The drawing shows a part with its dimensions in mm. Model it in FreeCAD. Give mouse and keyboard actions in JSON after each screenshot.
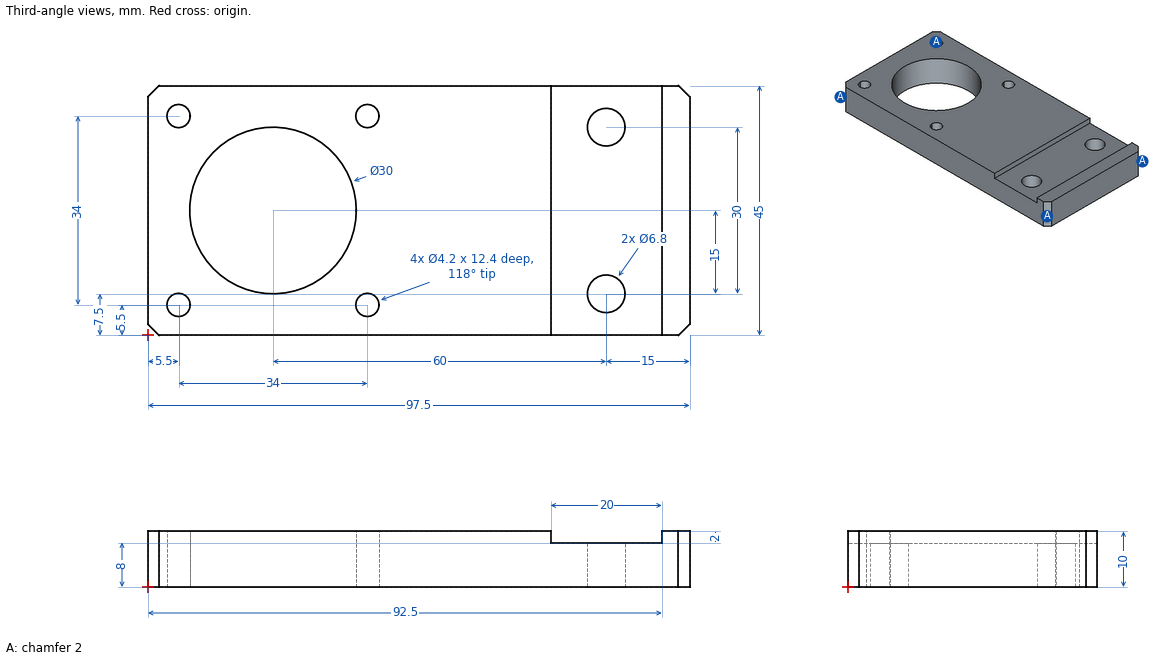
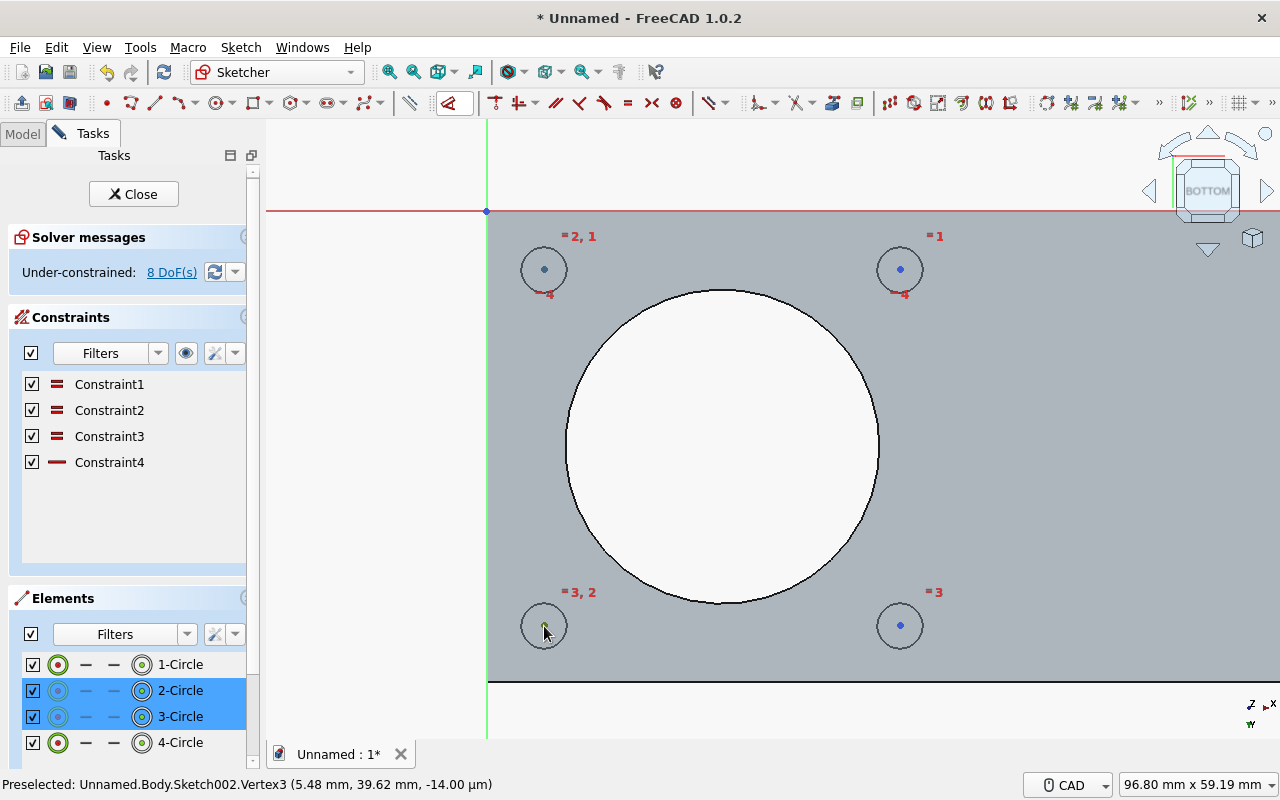
{"action": "left_click", "coordinate": [538, 104]}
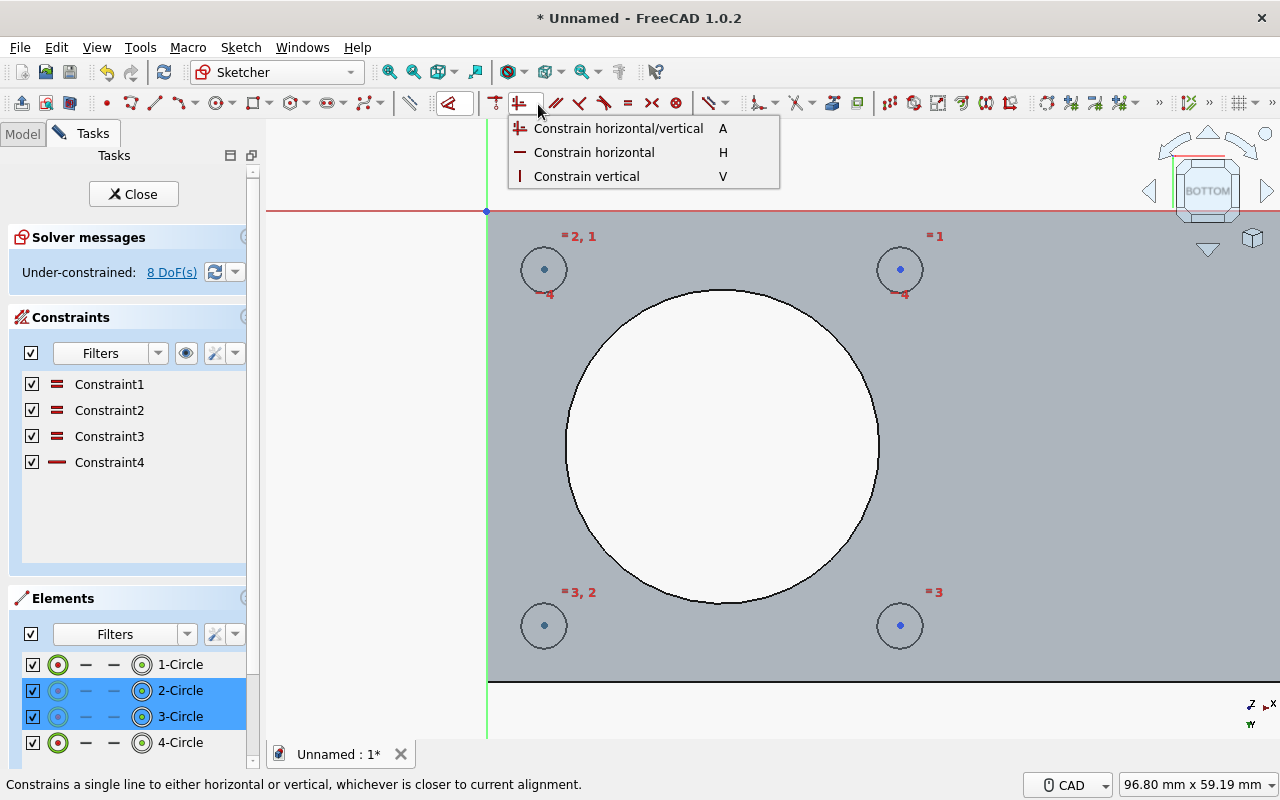
{"action": "left_click", "coordinate": [644, 176]}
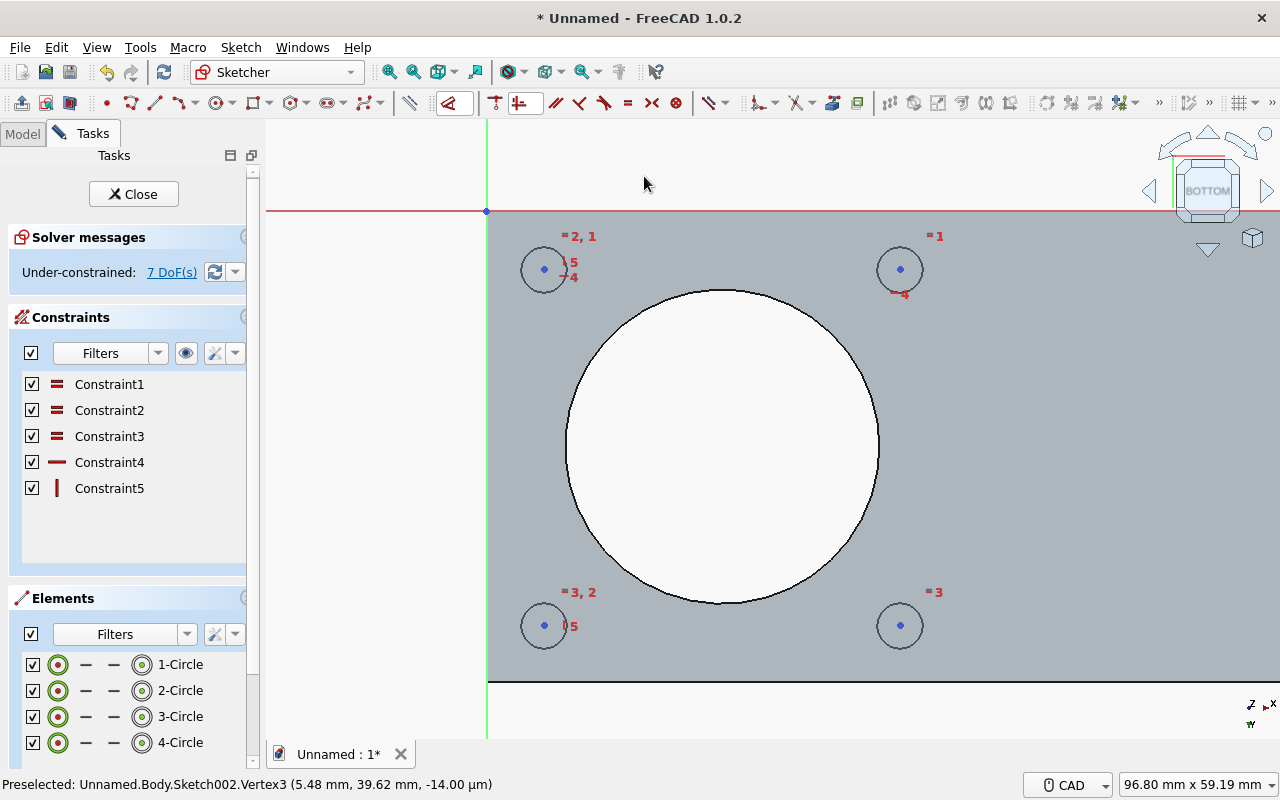
{"action": "left_click", "coordinate": [900, 270]}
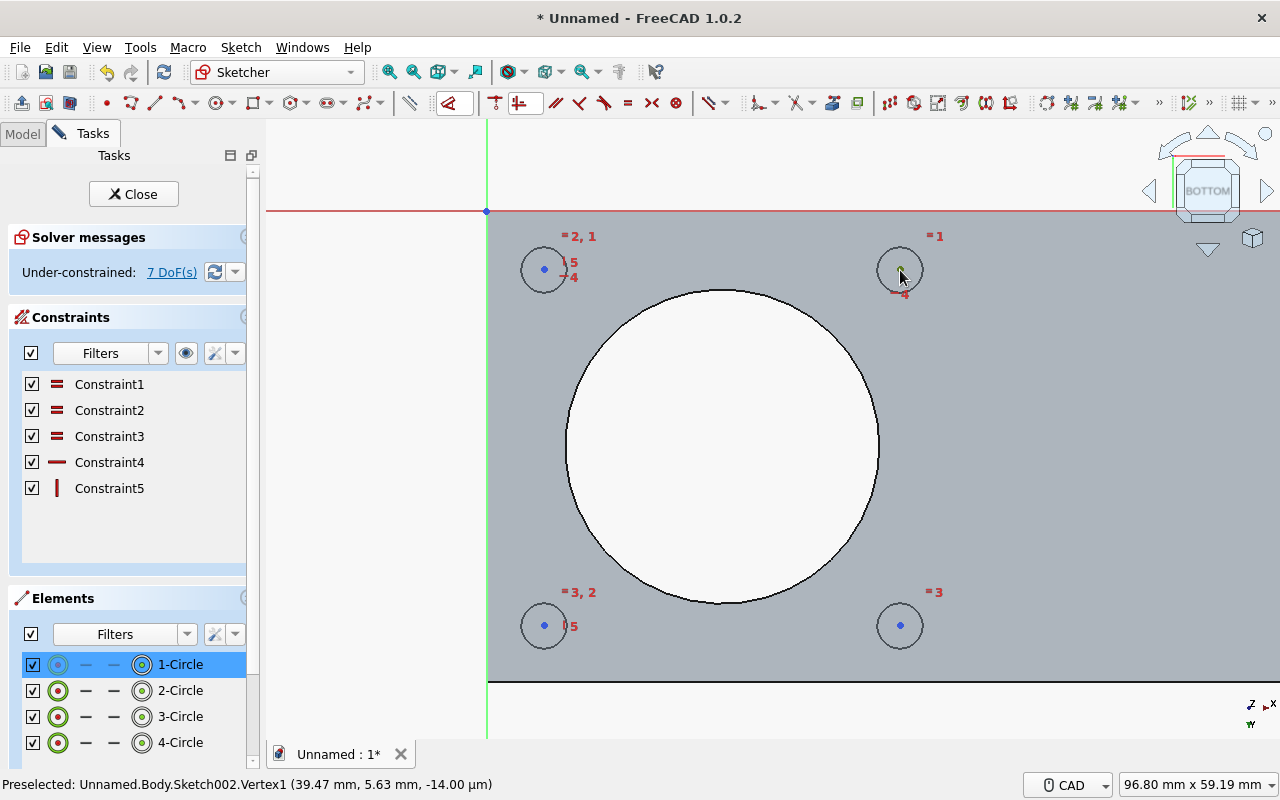
{"action": "left_click", "coordinate": [900, 626]}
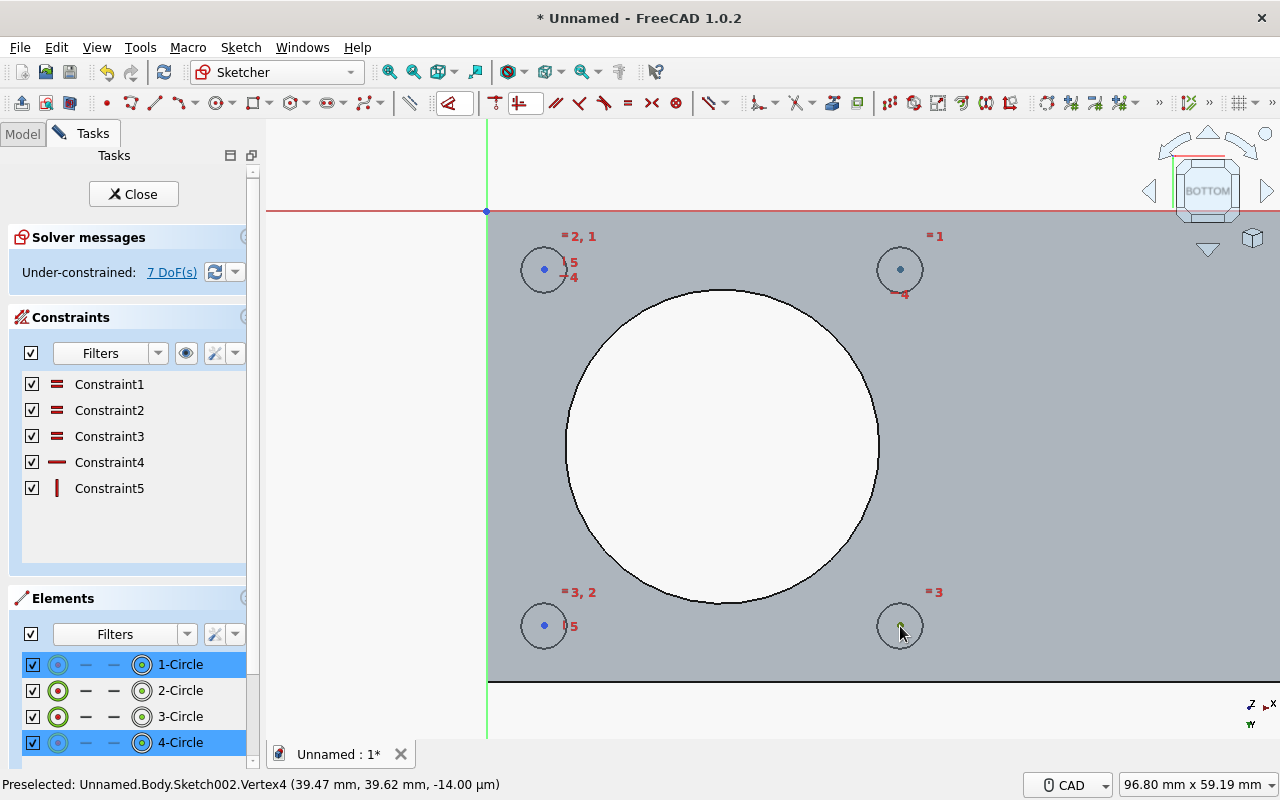
{"action": "left_click", "coordinate": [538, 104]}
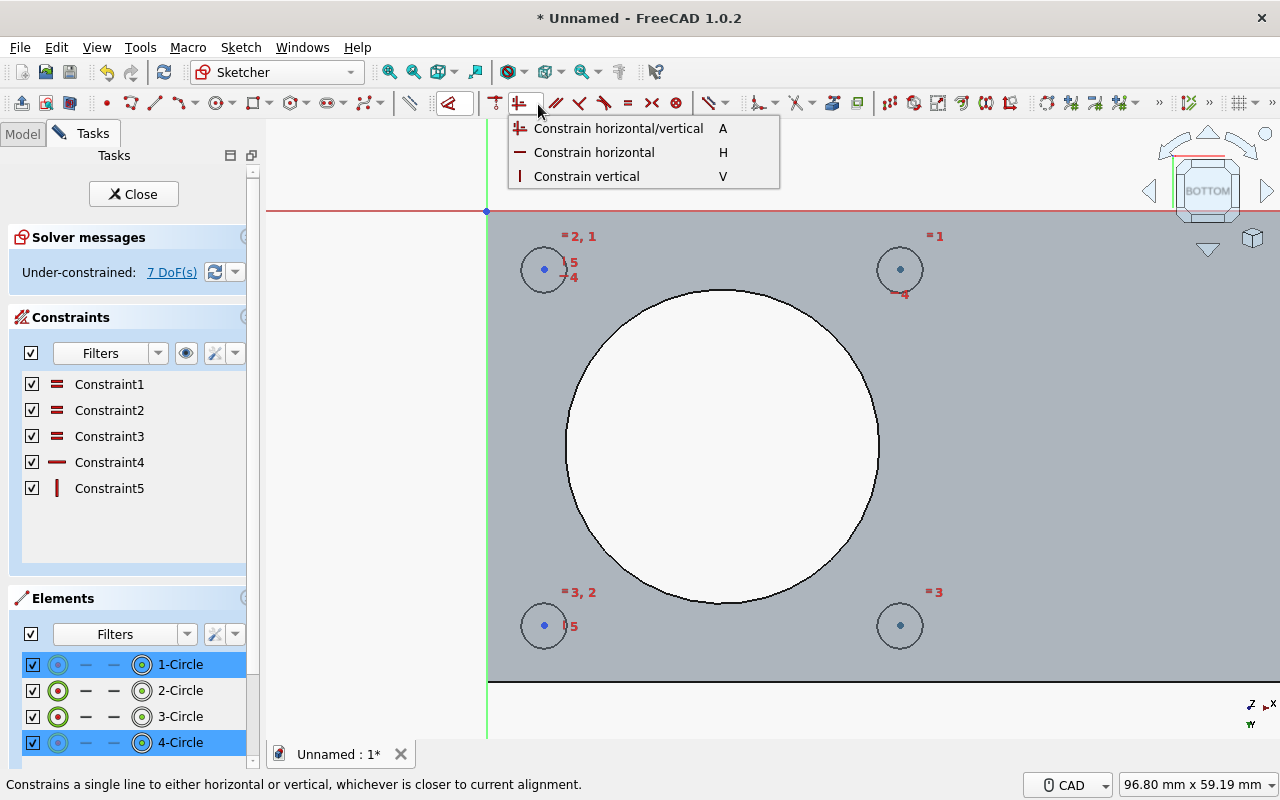
{"action": "left_click", "coordinate": [644, 176]}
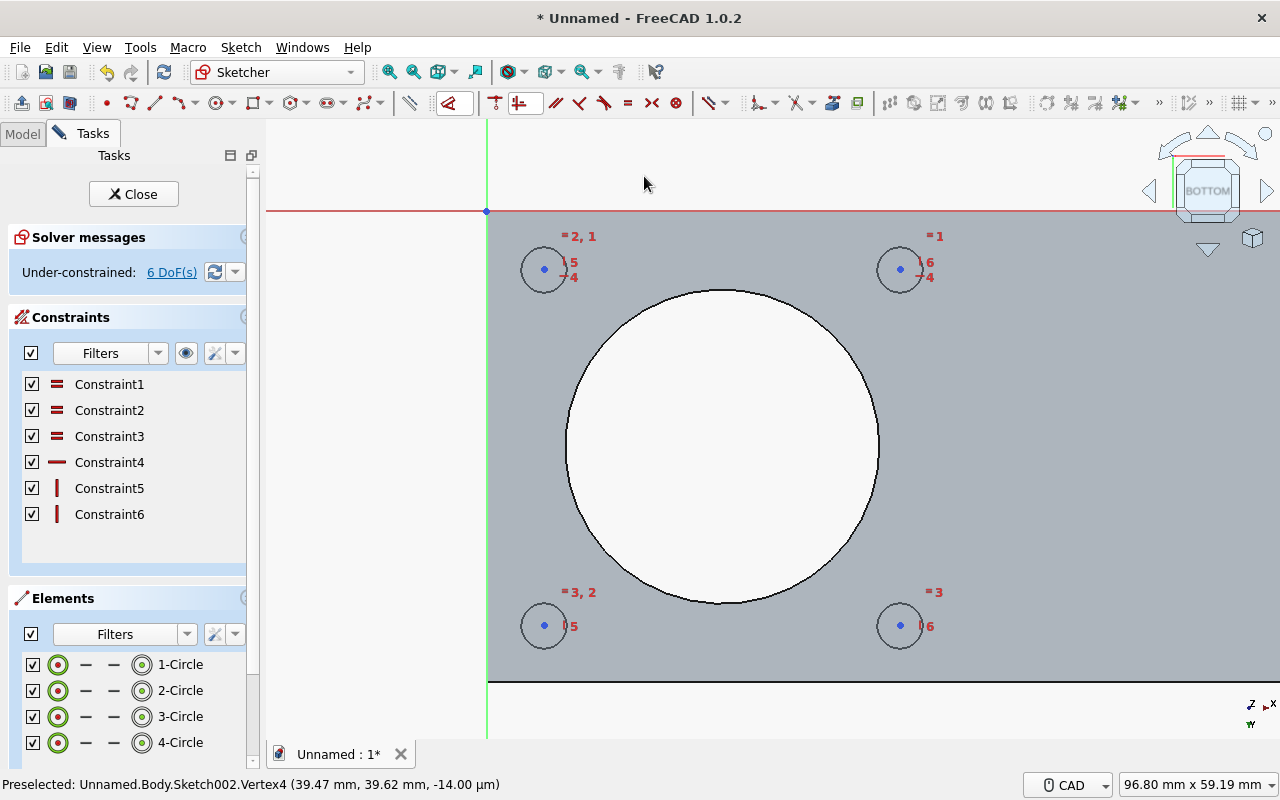
{"action": "left_click", "coordinate": [544, 626]}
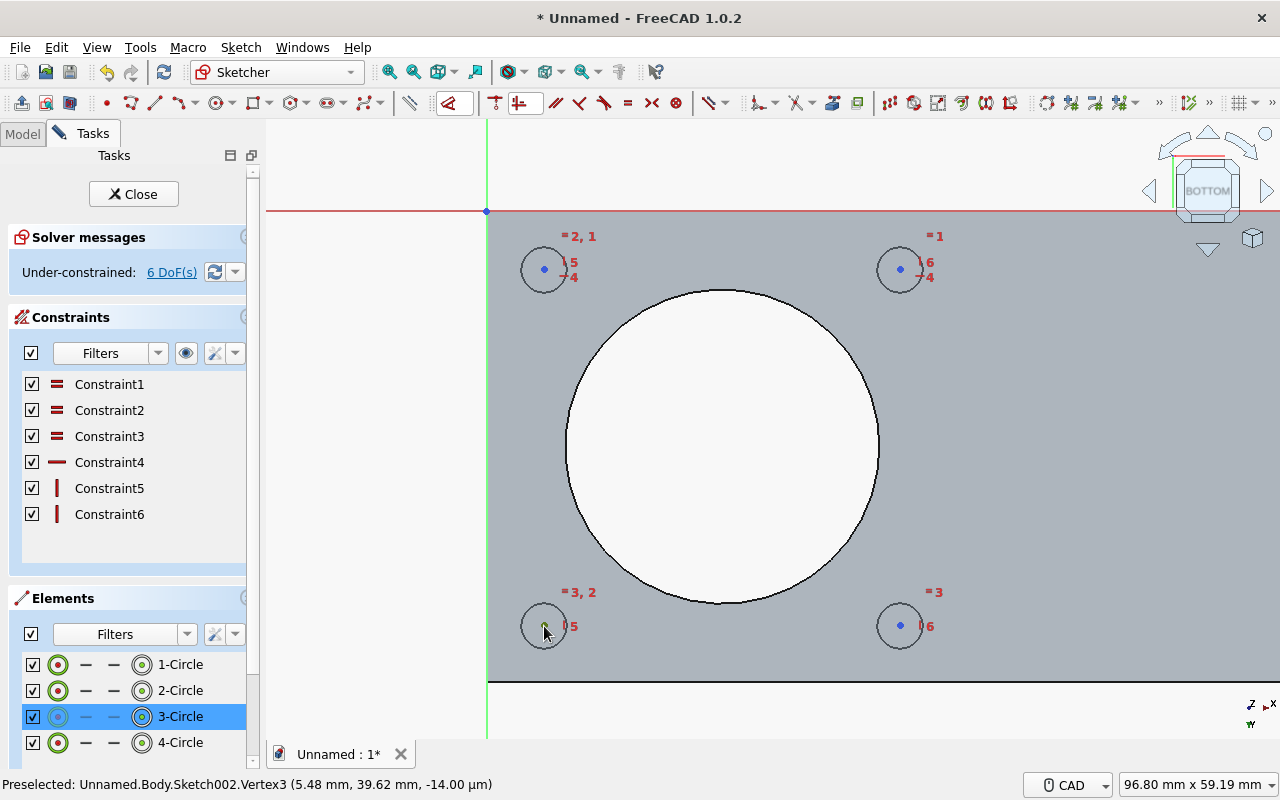
{"action": "left_click", "coordinate": [900, 626]}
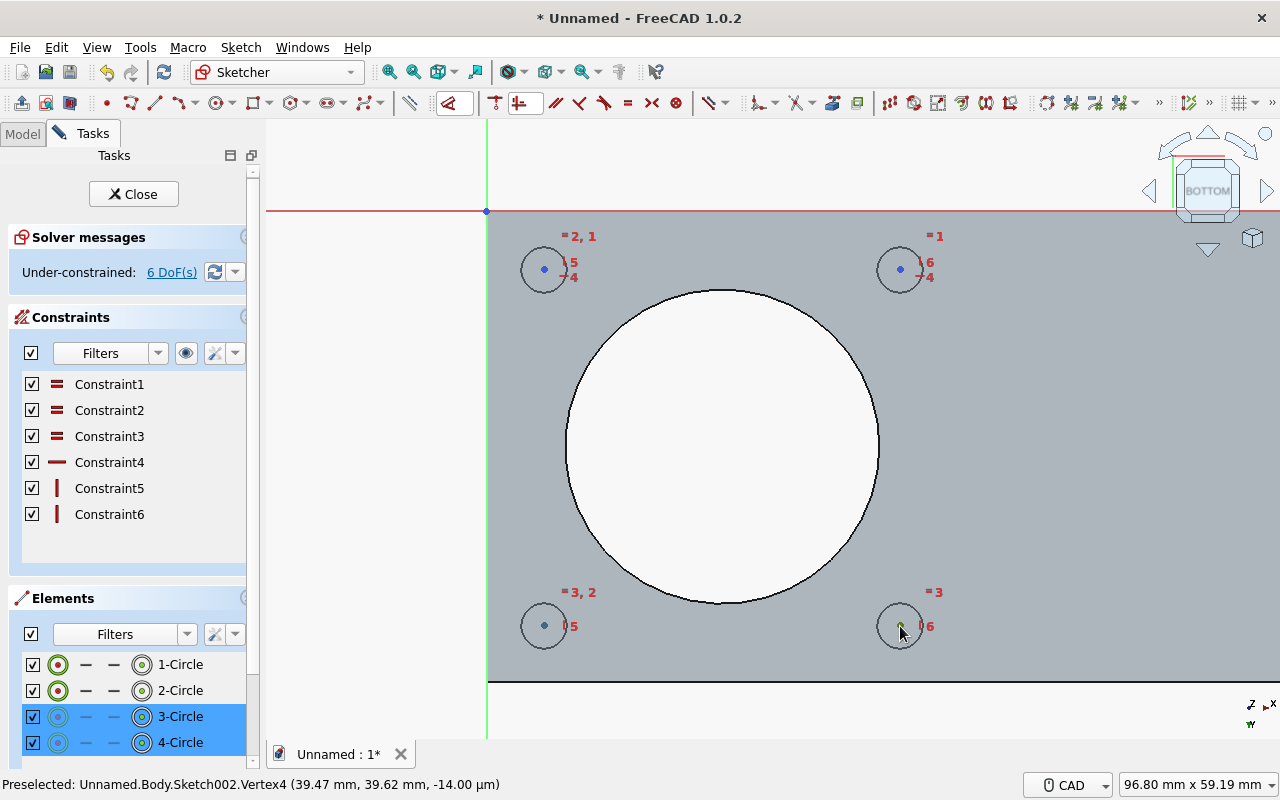
{"action": "key", "text": "h"}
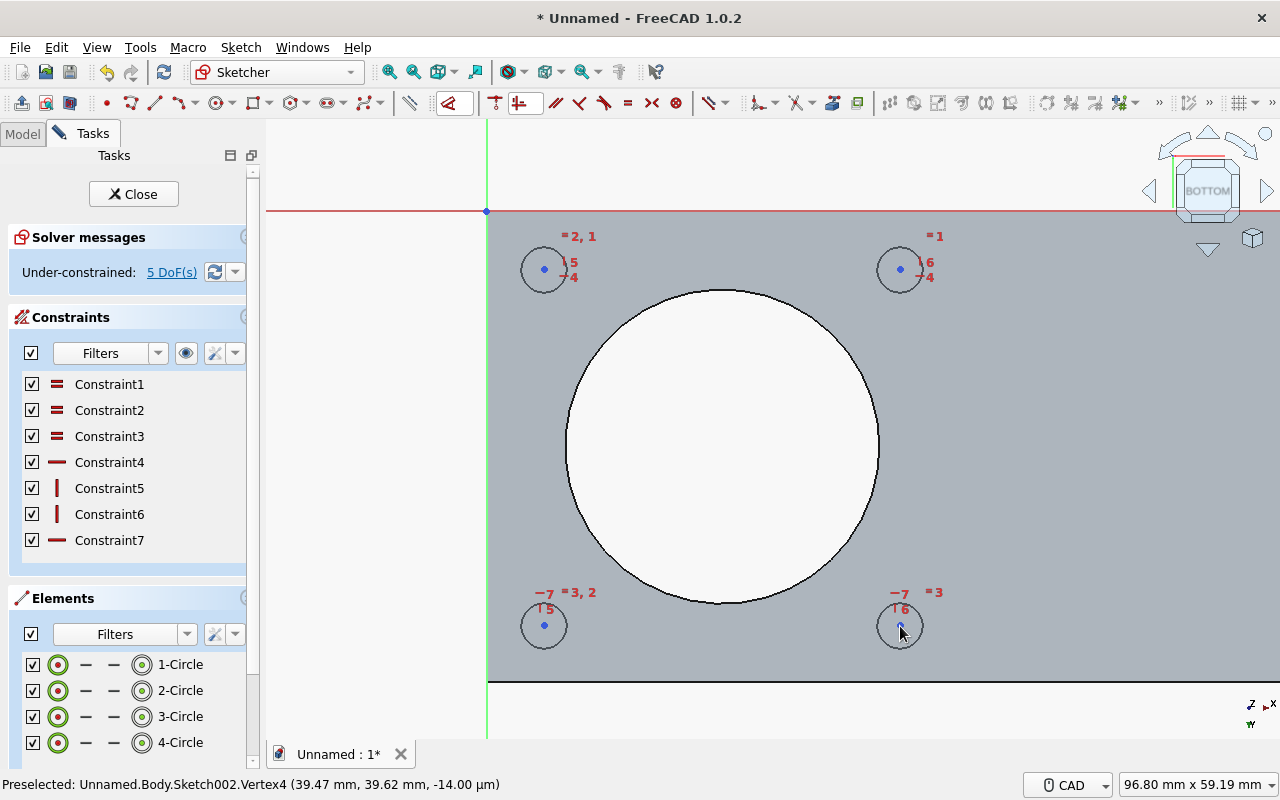
{"action": "left_click", "coordinate": [884, 254]}